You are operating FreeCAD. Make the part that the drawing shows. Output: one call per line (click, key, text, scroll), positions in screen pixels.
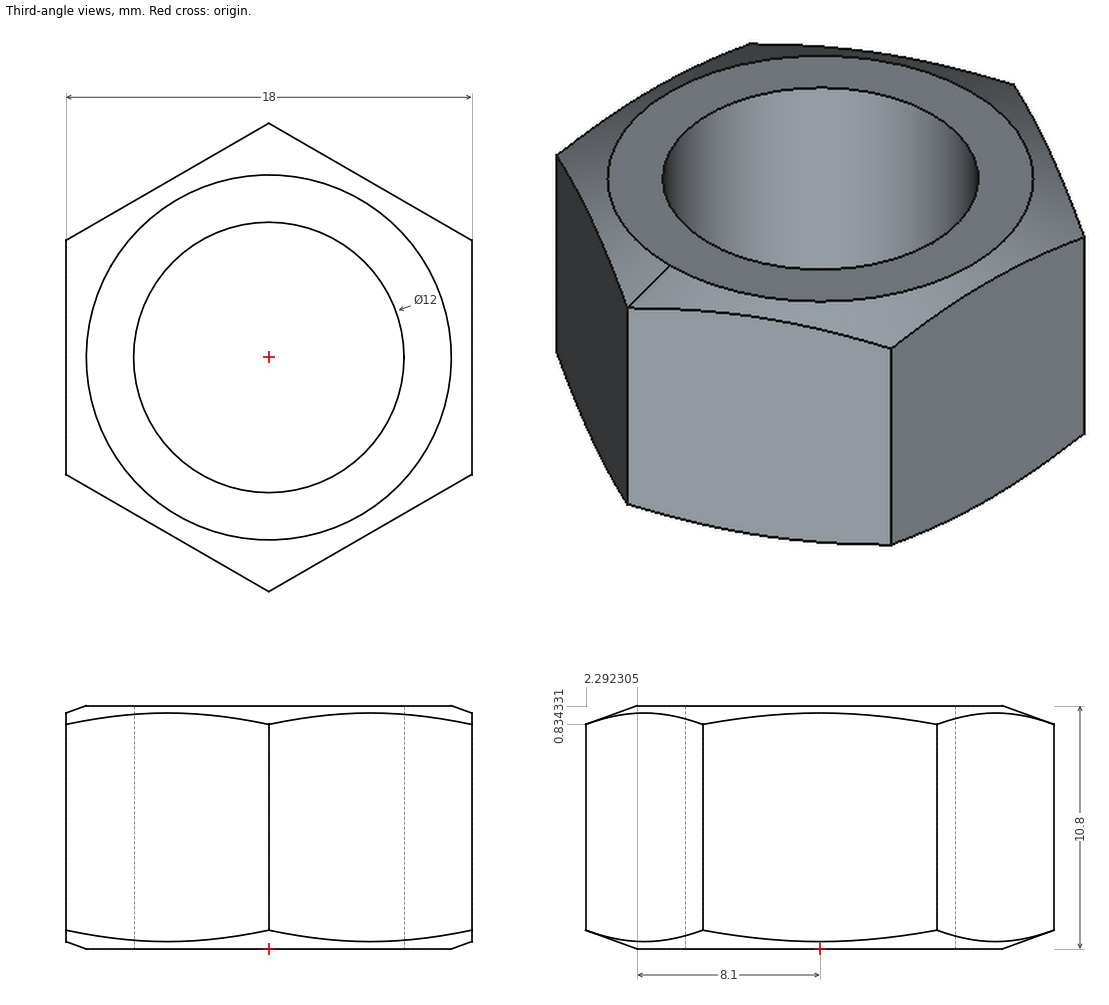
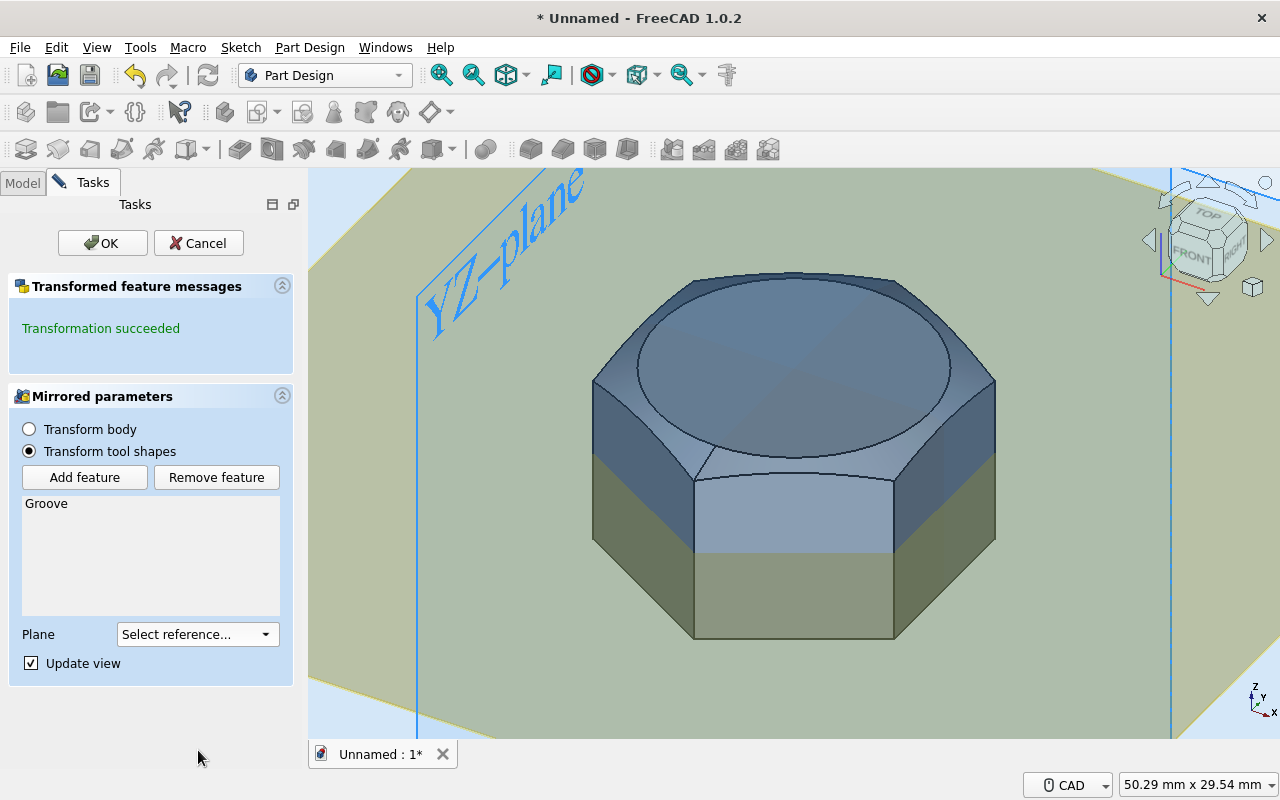
click(23, 182)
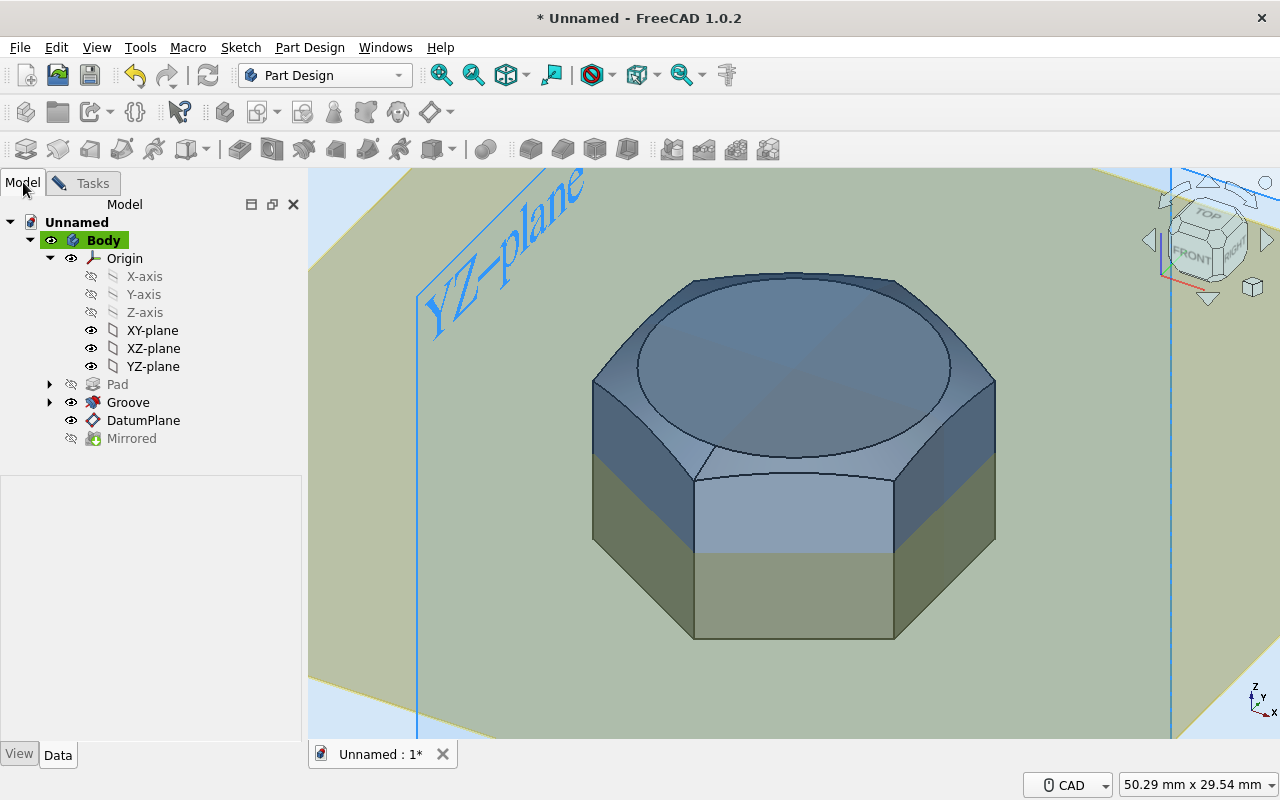
click(116, 420)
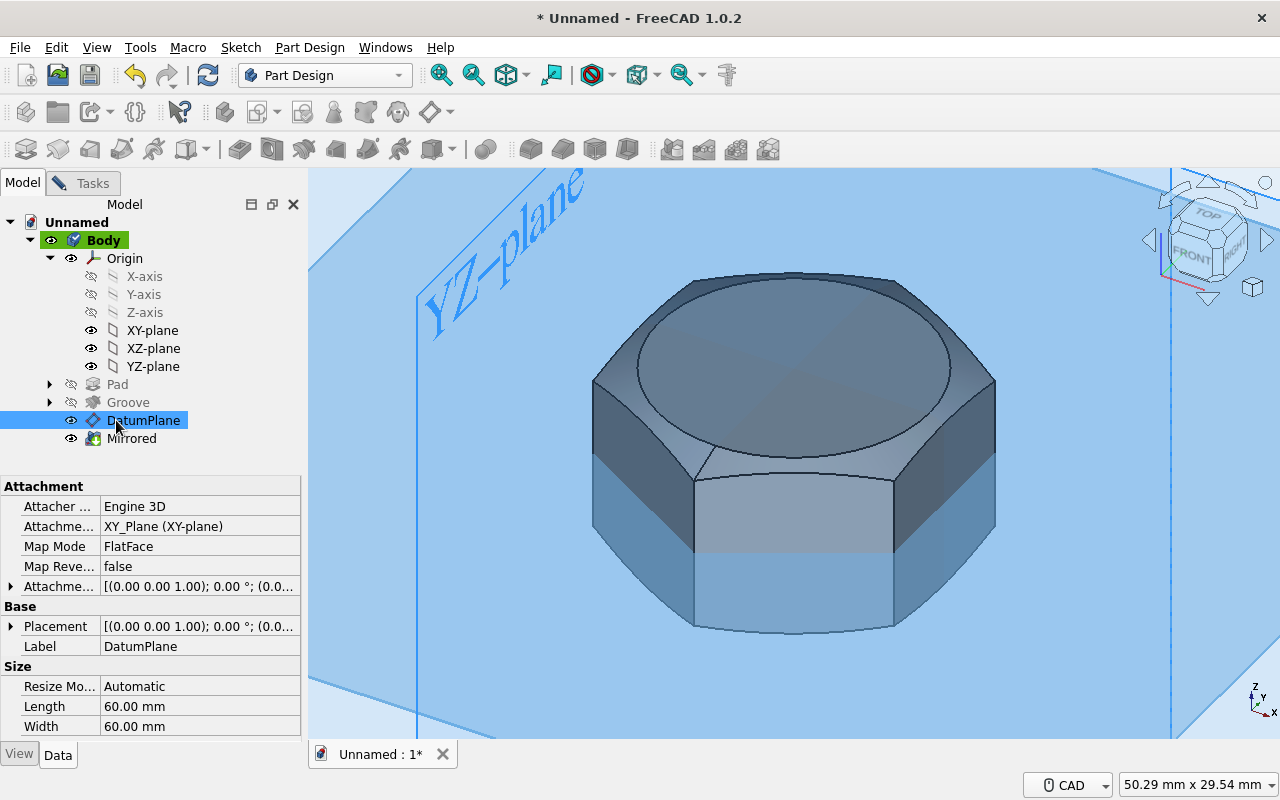
click(84, 182)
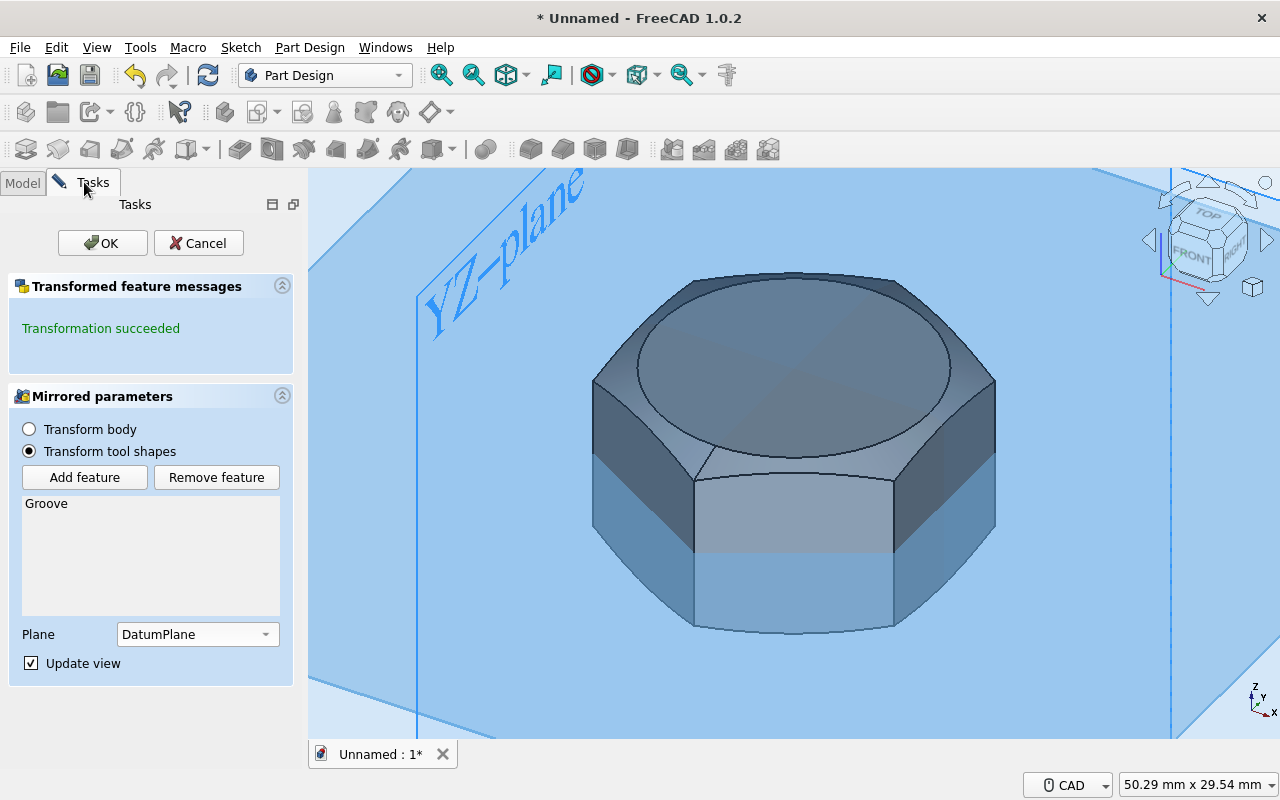
click(103, 243)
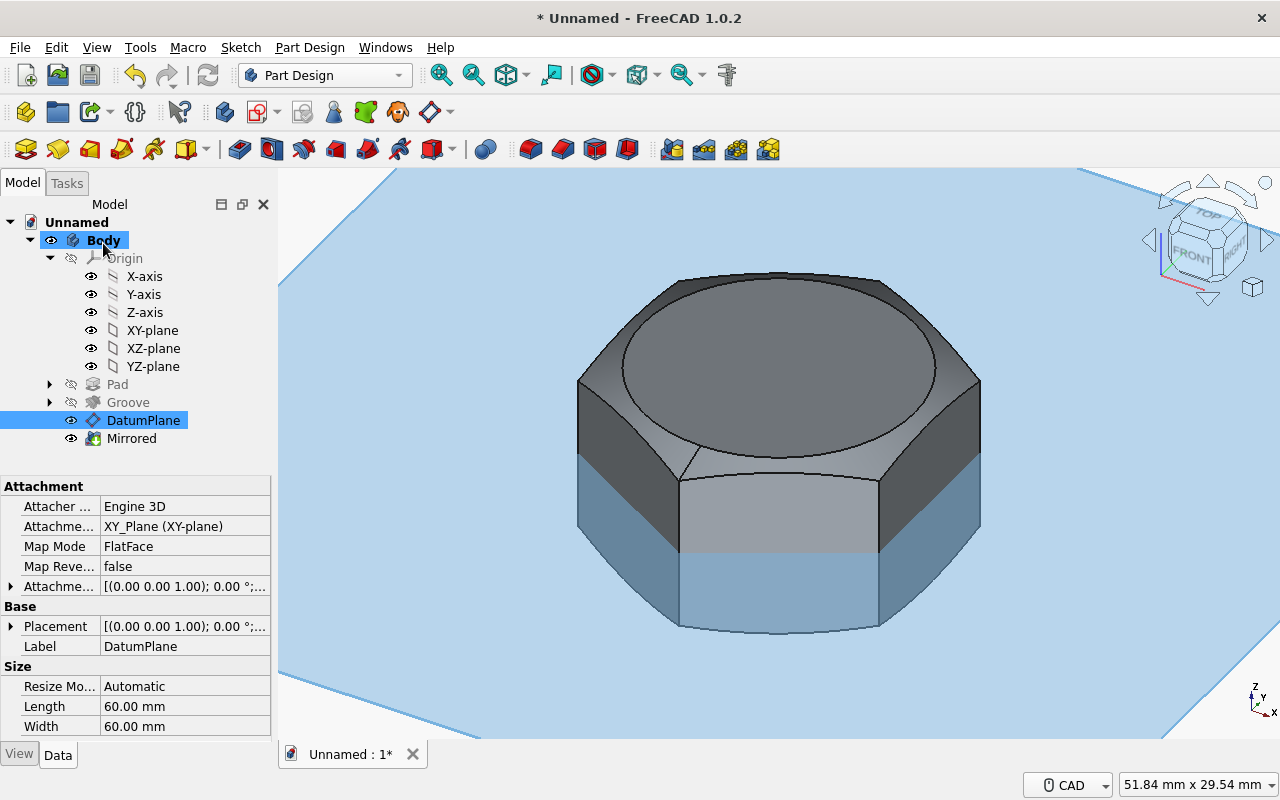
click(116, 420)
key(space)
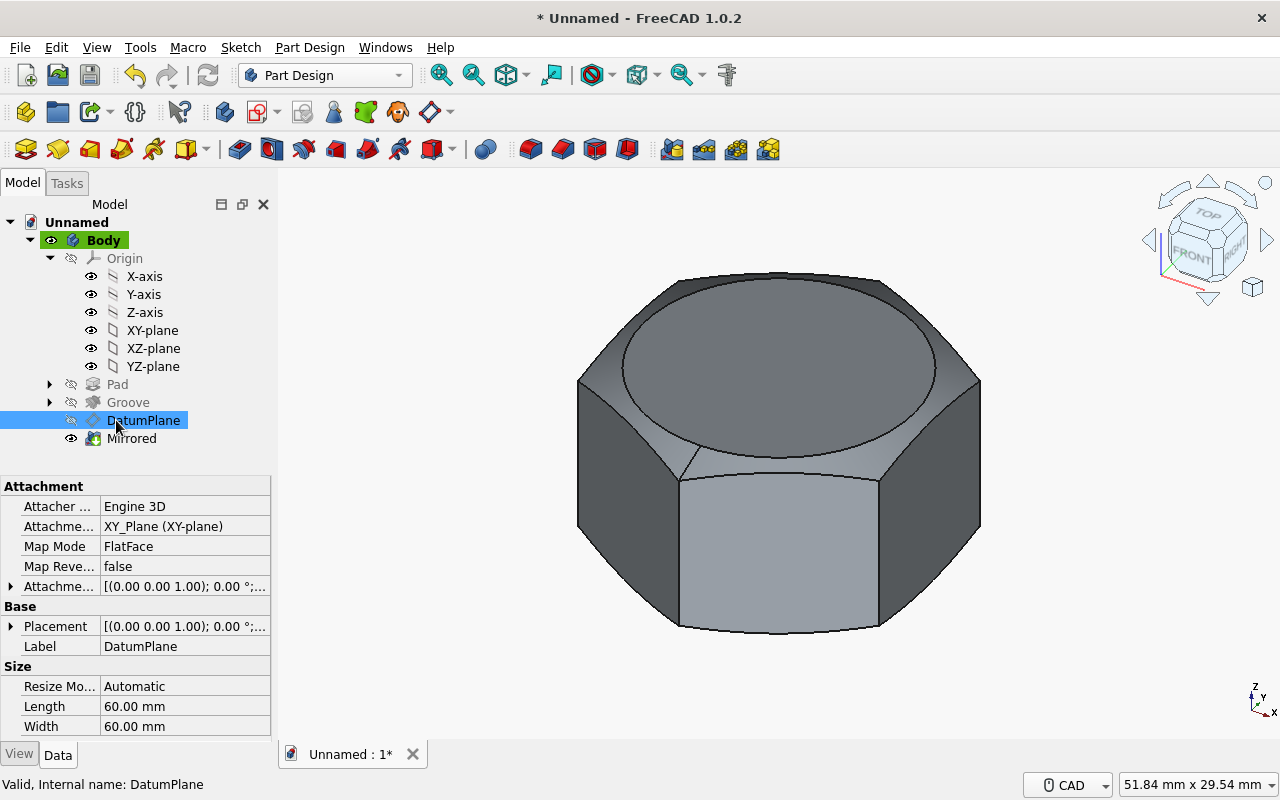
click(779, 367)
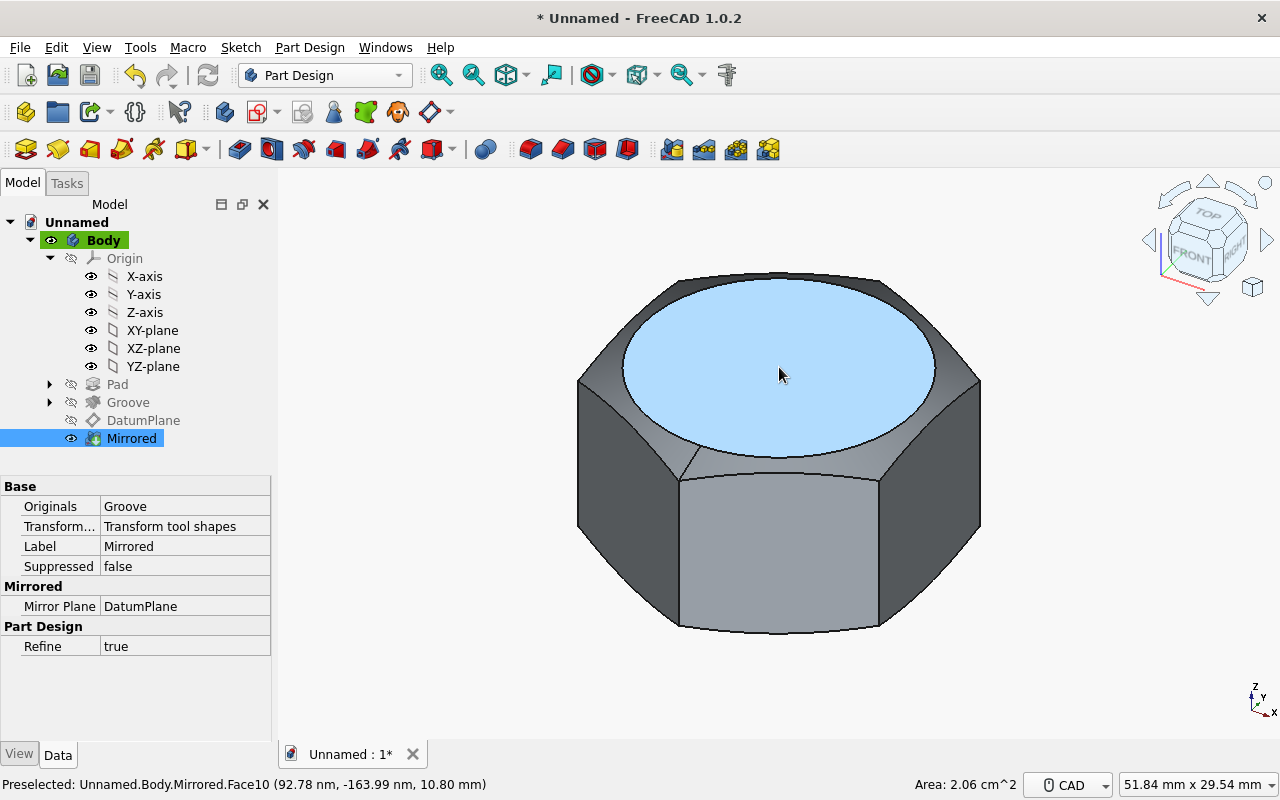
click(258, 112)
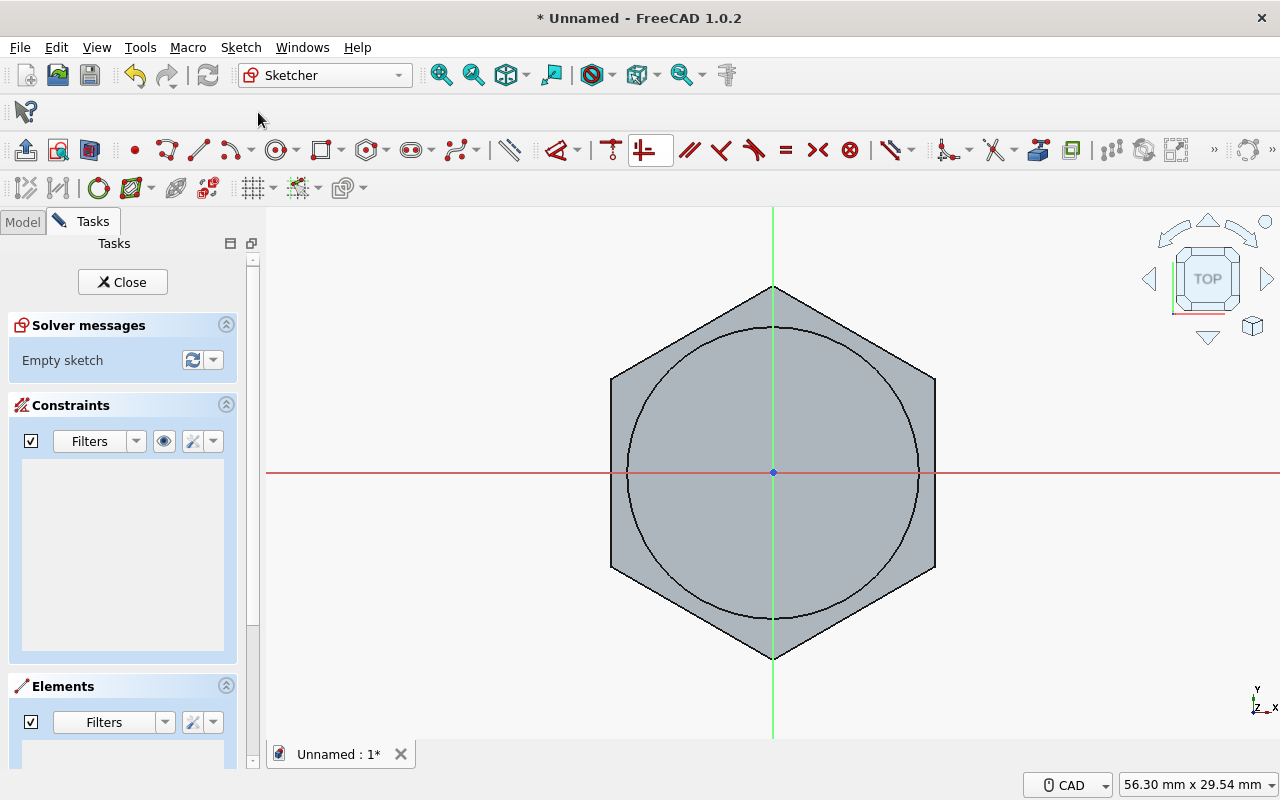
scroll(912, 473, up, 2)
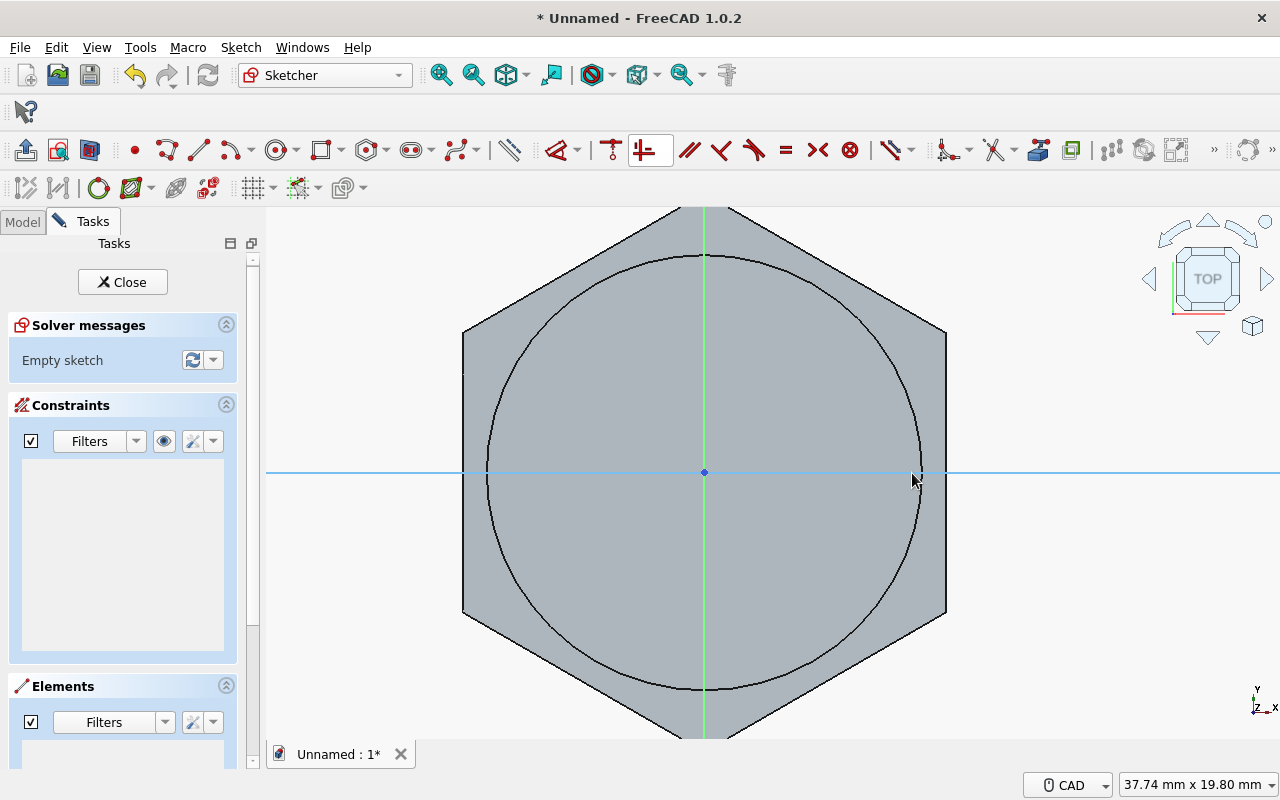
click(276, 150)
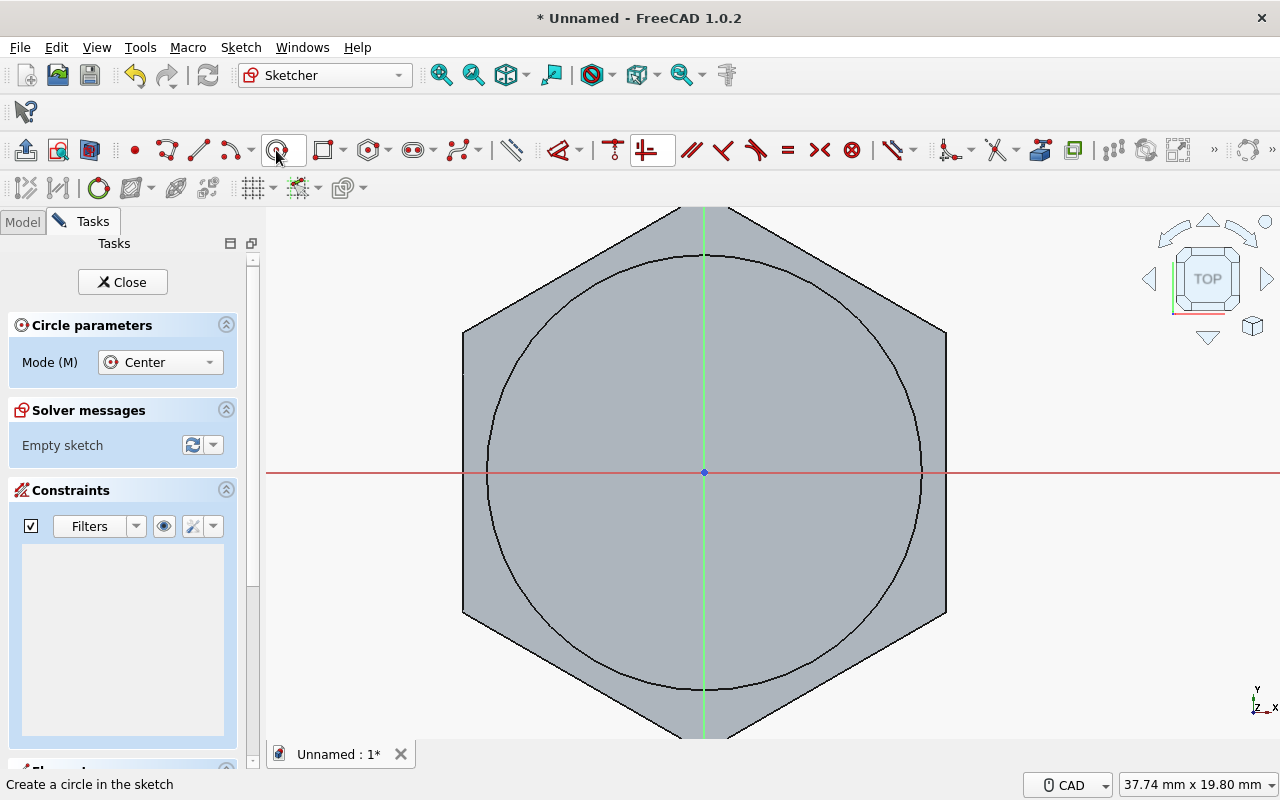
click(704, 473)
move(818, 359)